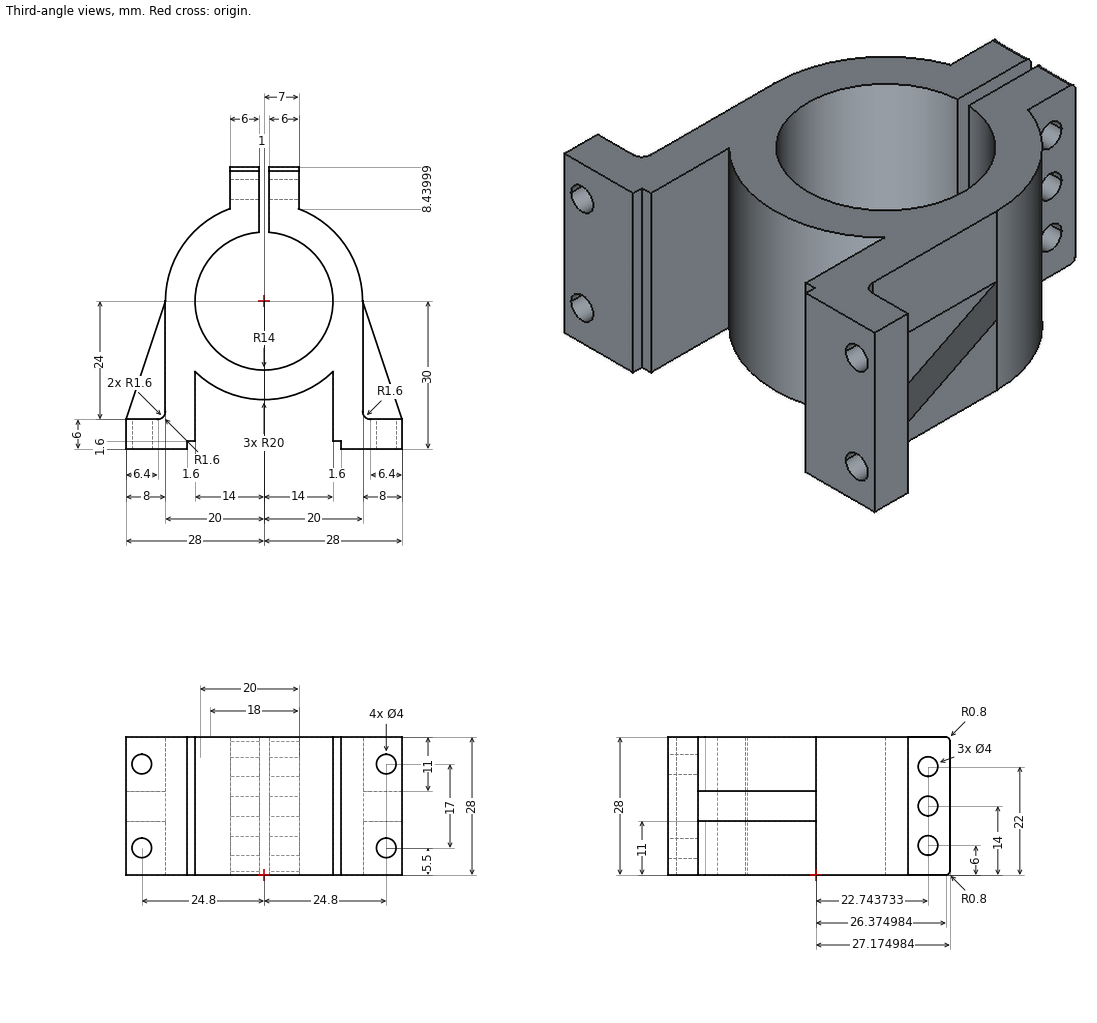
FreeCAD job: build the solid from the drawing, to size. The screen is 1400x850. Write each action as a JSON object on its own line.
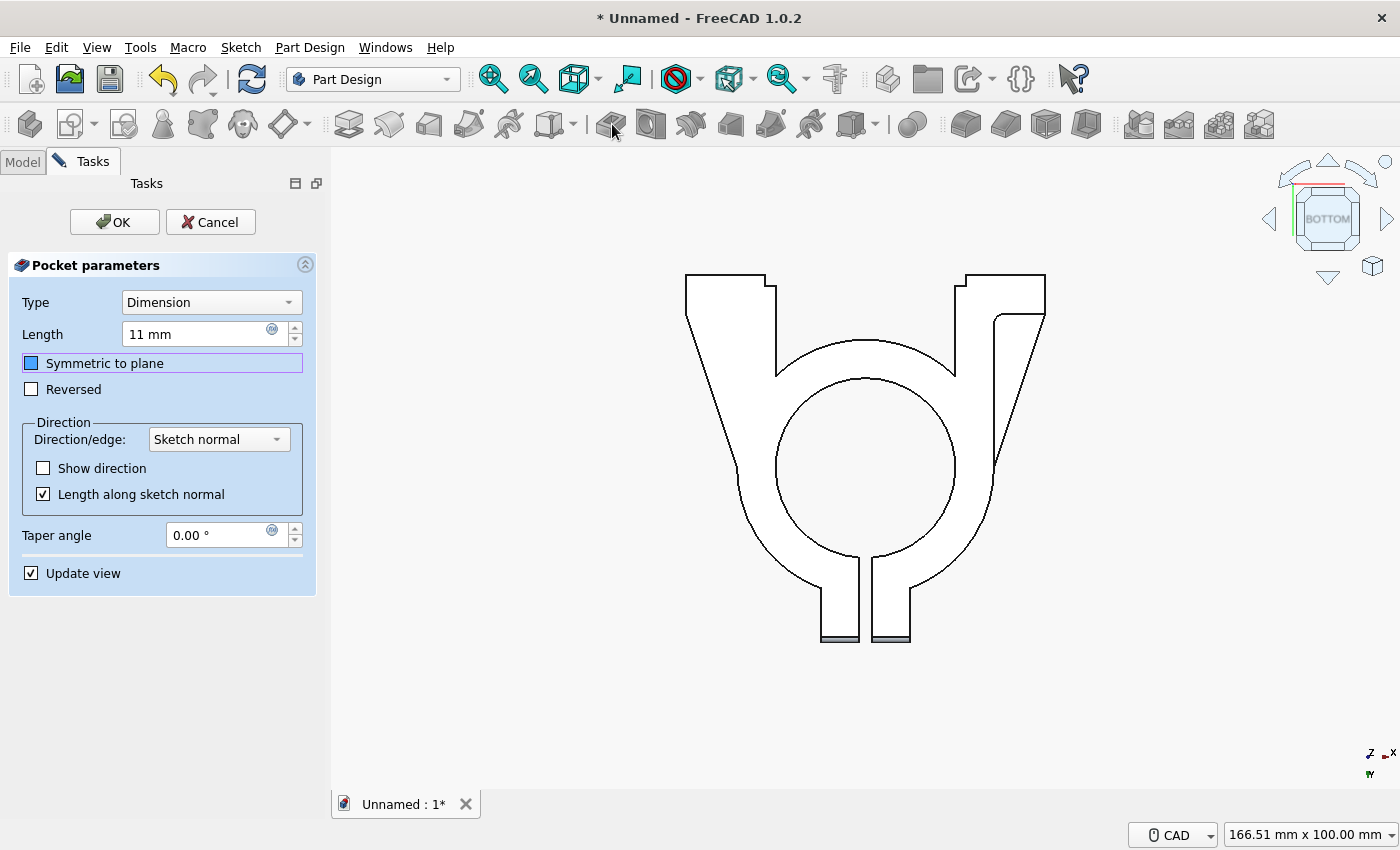
{"action": "left_click", "coordinate": [30, 389]}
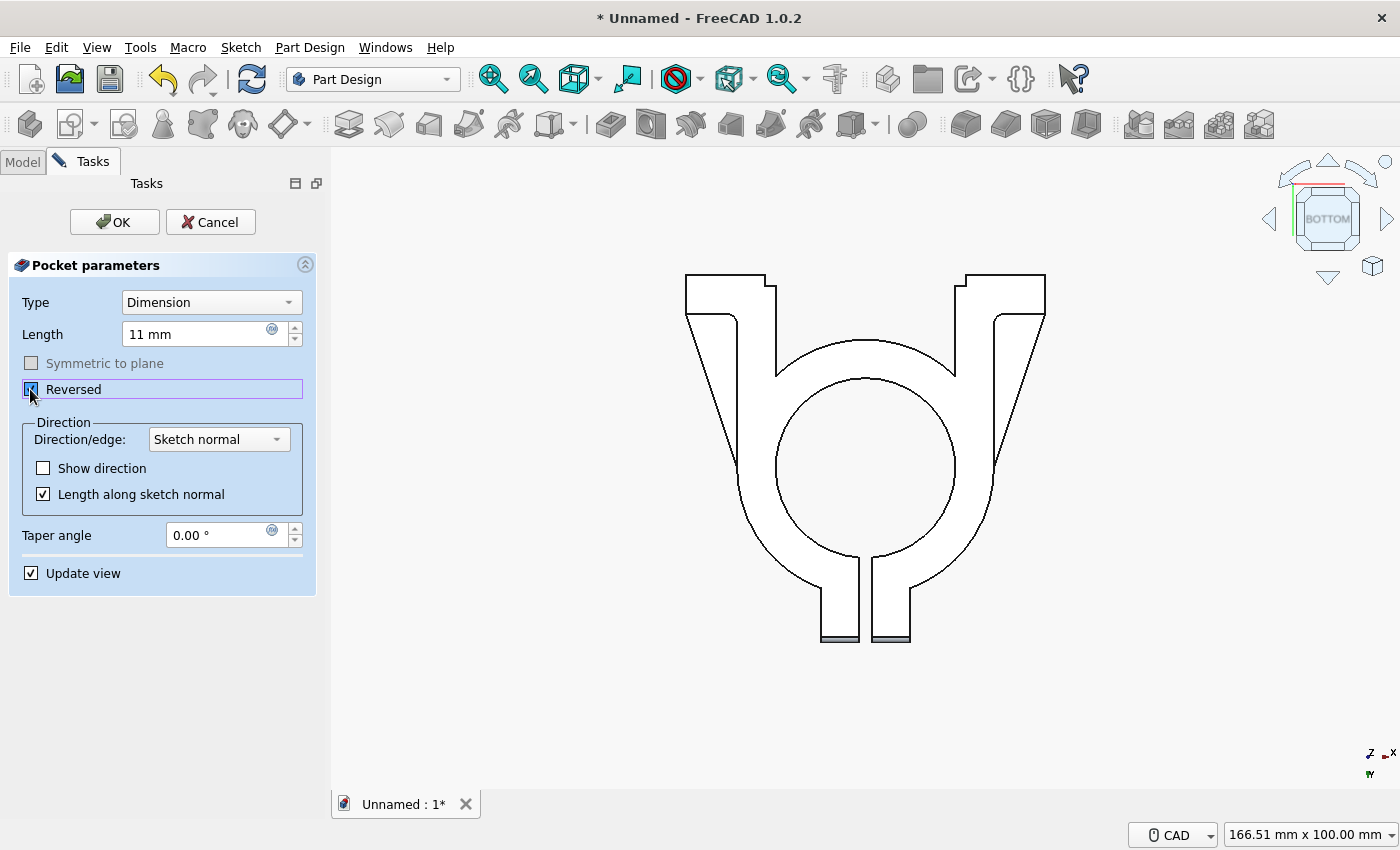
{"action": "left_click", "coordinate": [115, 222]}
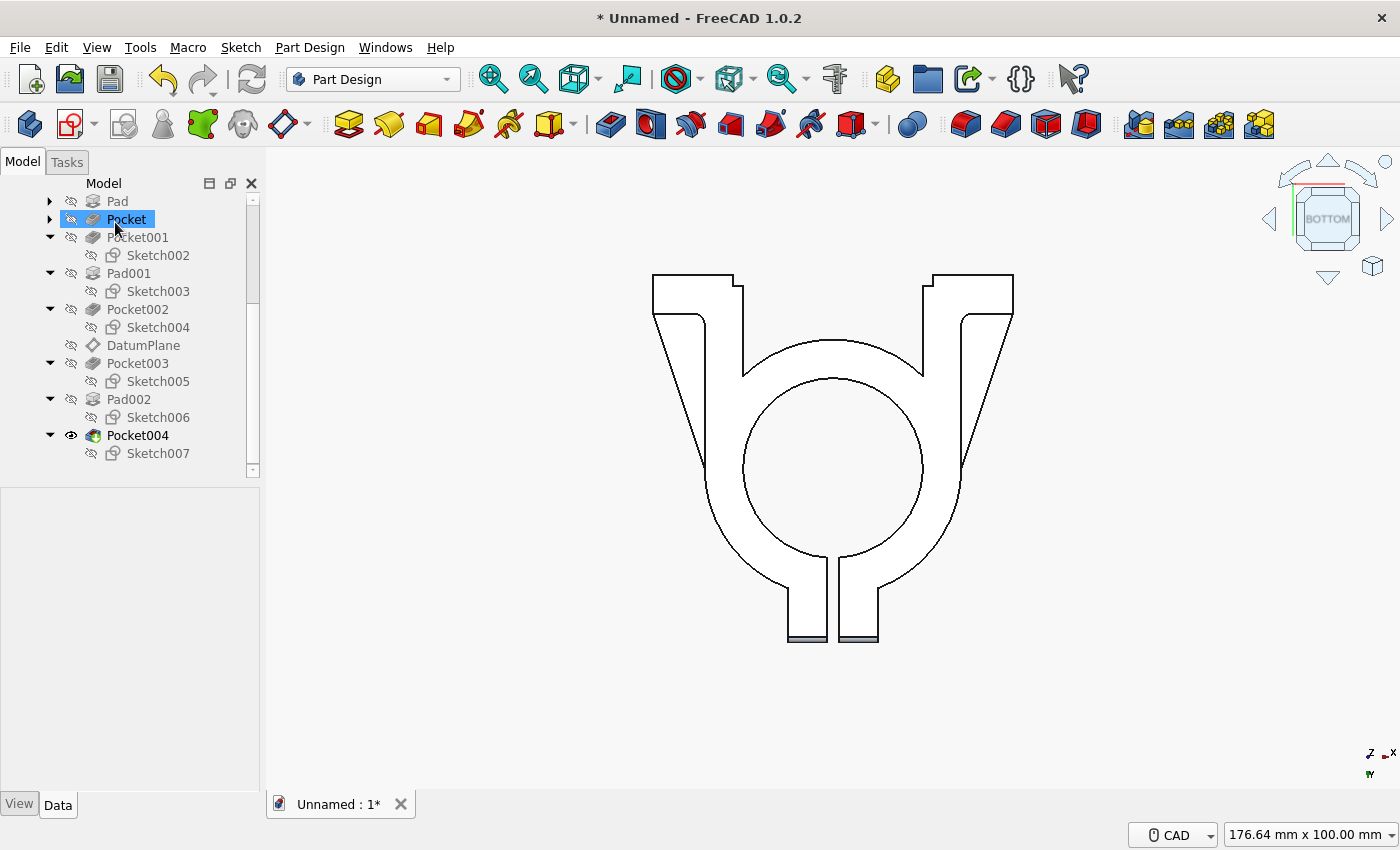
{"action": "key", "text": "0"}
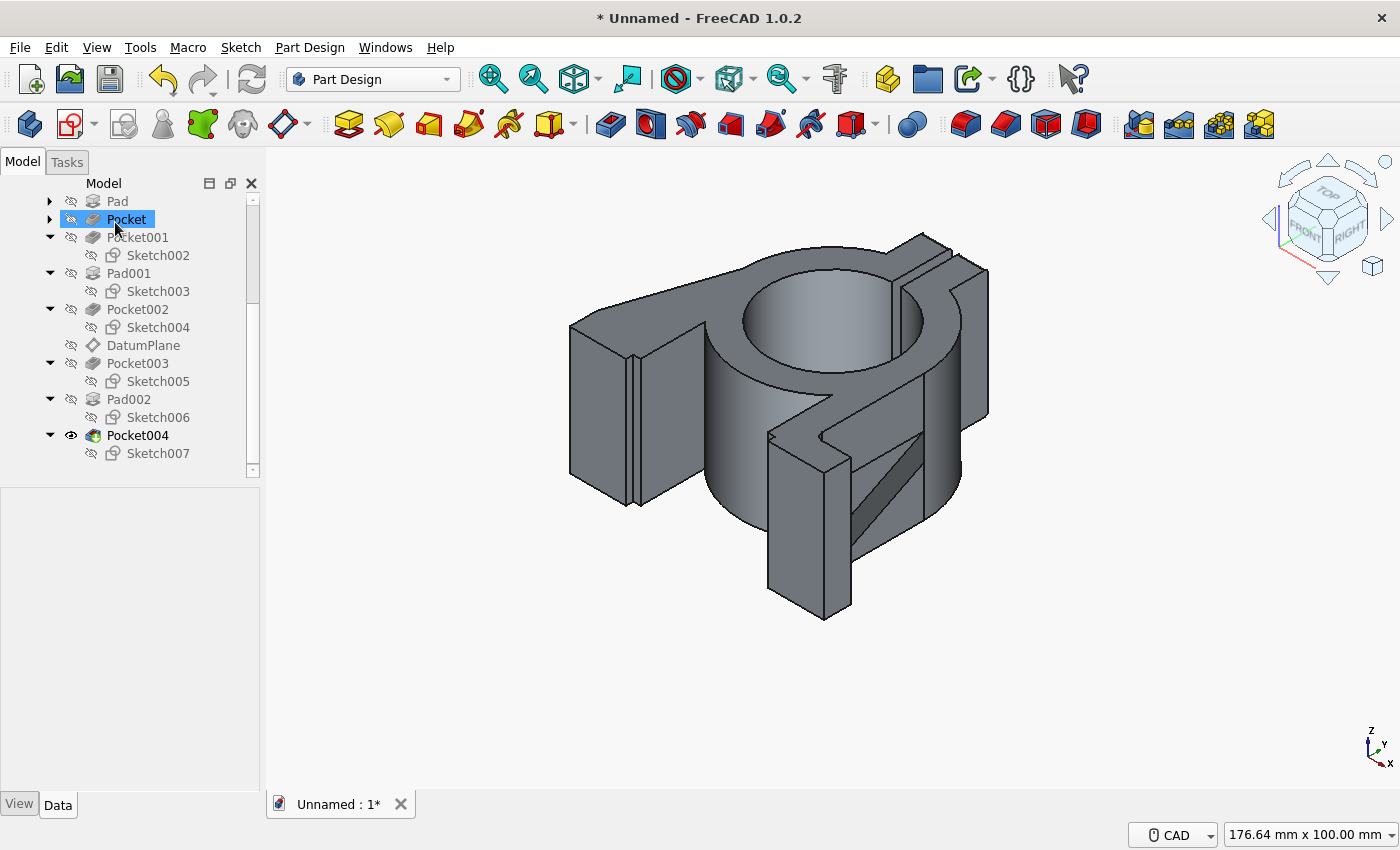
{"action": "left_click", "coordinate": [867, 478]}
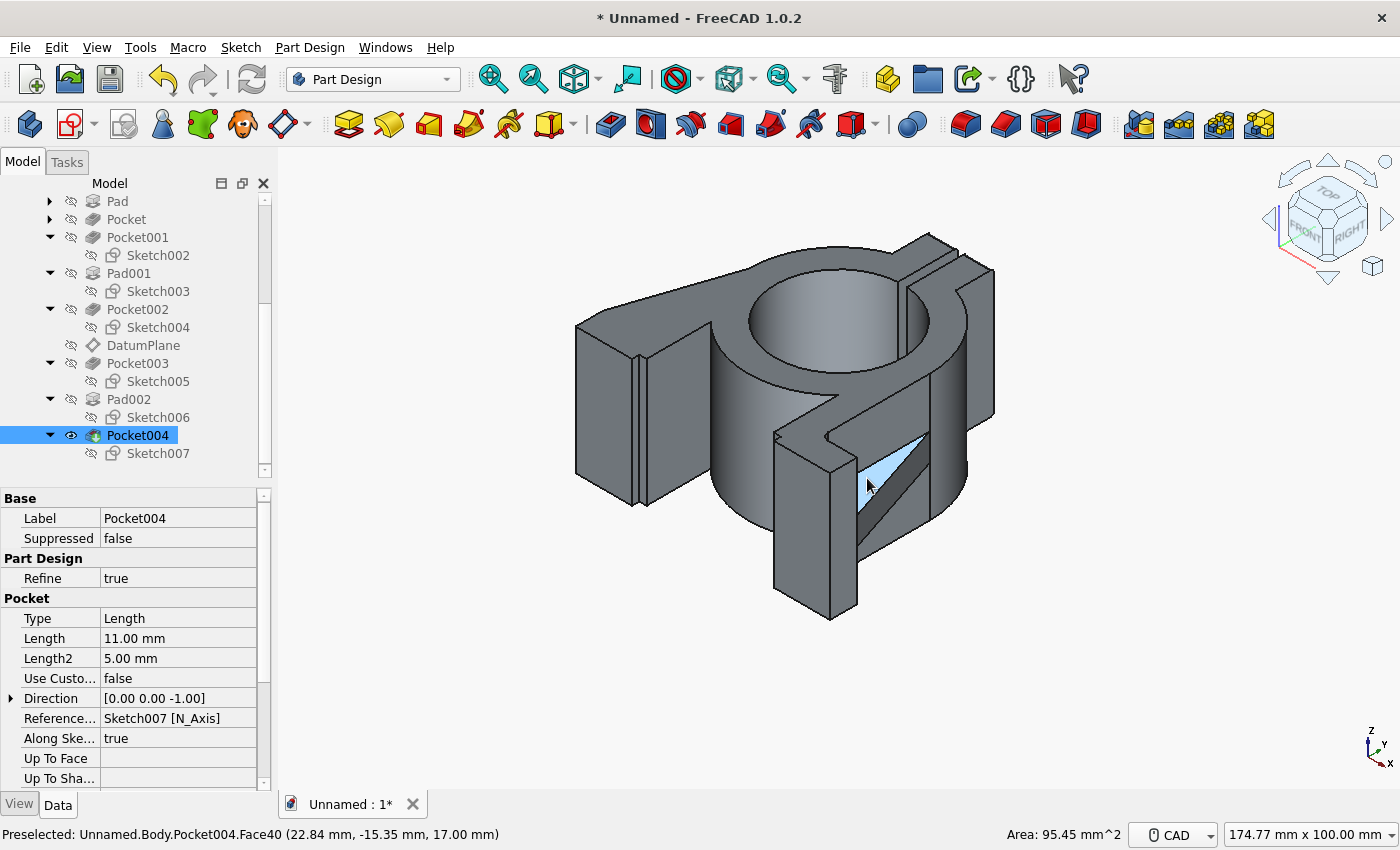
{"action": "left_click", "coordinate": [70, 124]}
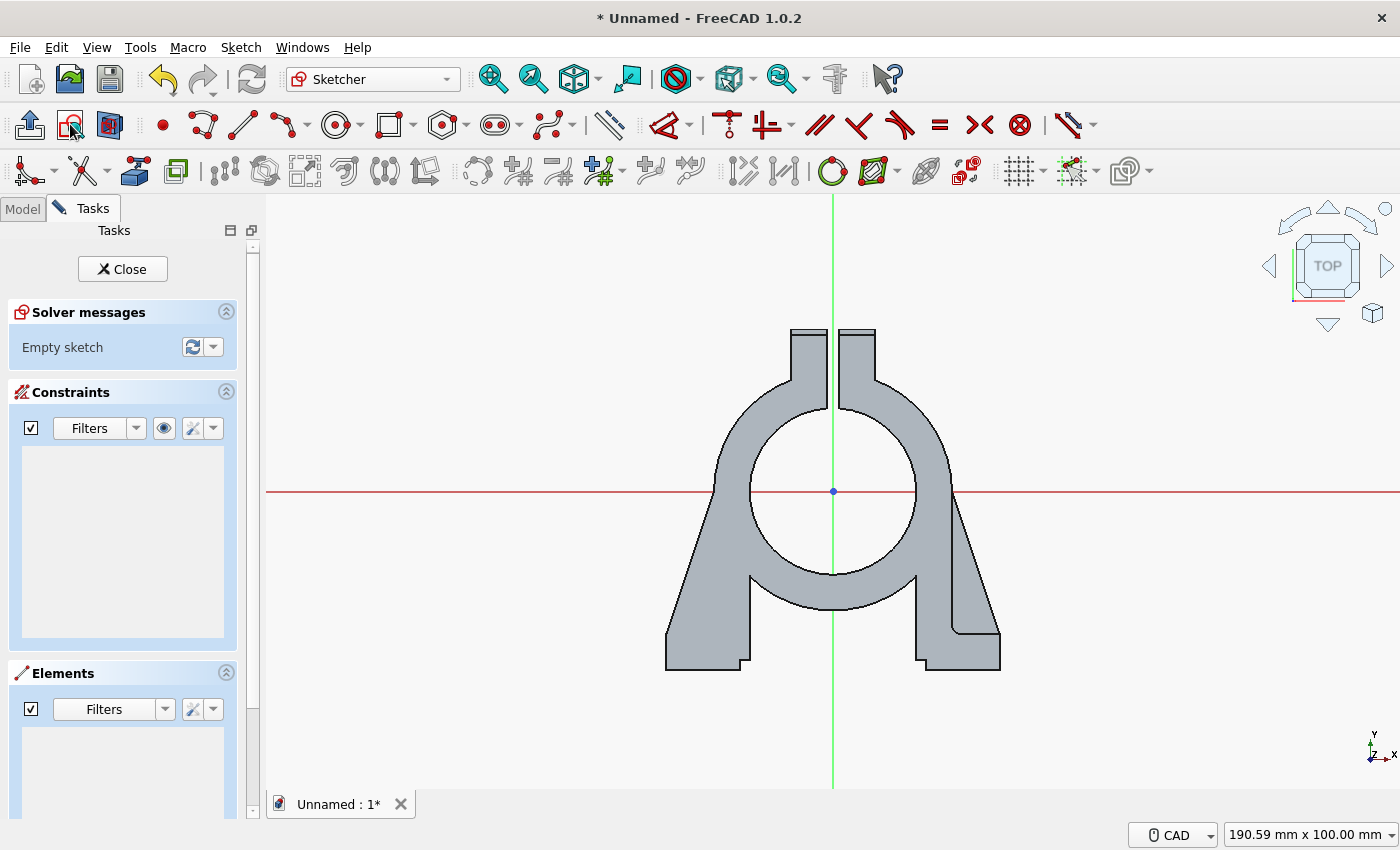
{"action": "scroll", "coordinate": [741, 604], "scroll_direction": "up", "scroll_amount": 5}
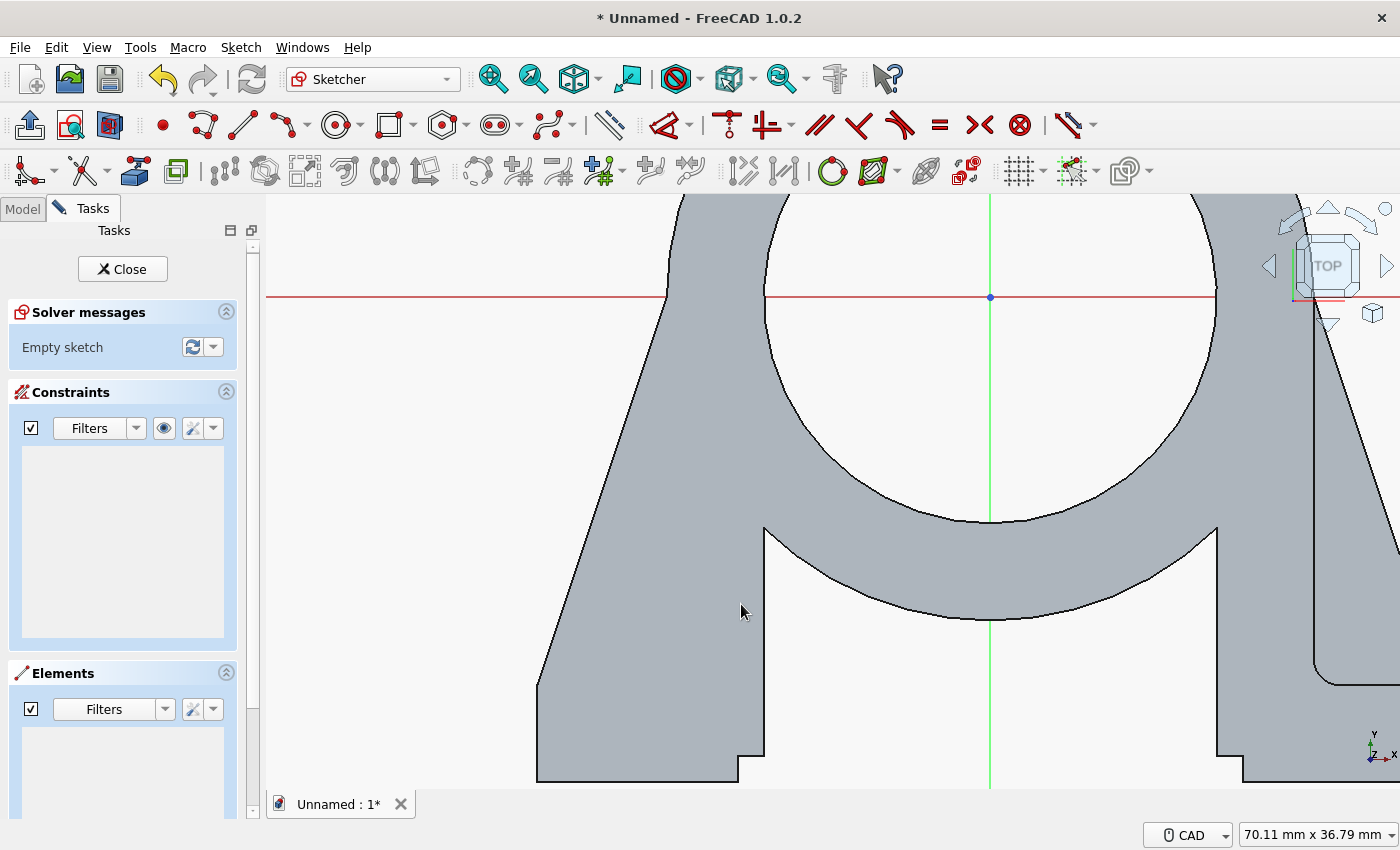
{"action": "left_click", "coordinate": [204, 126]}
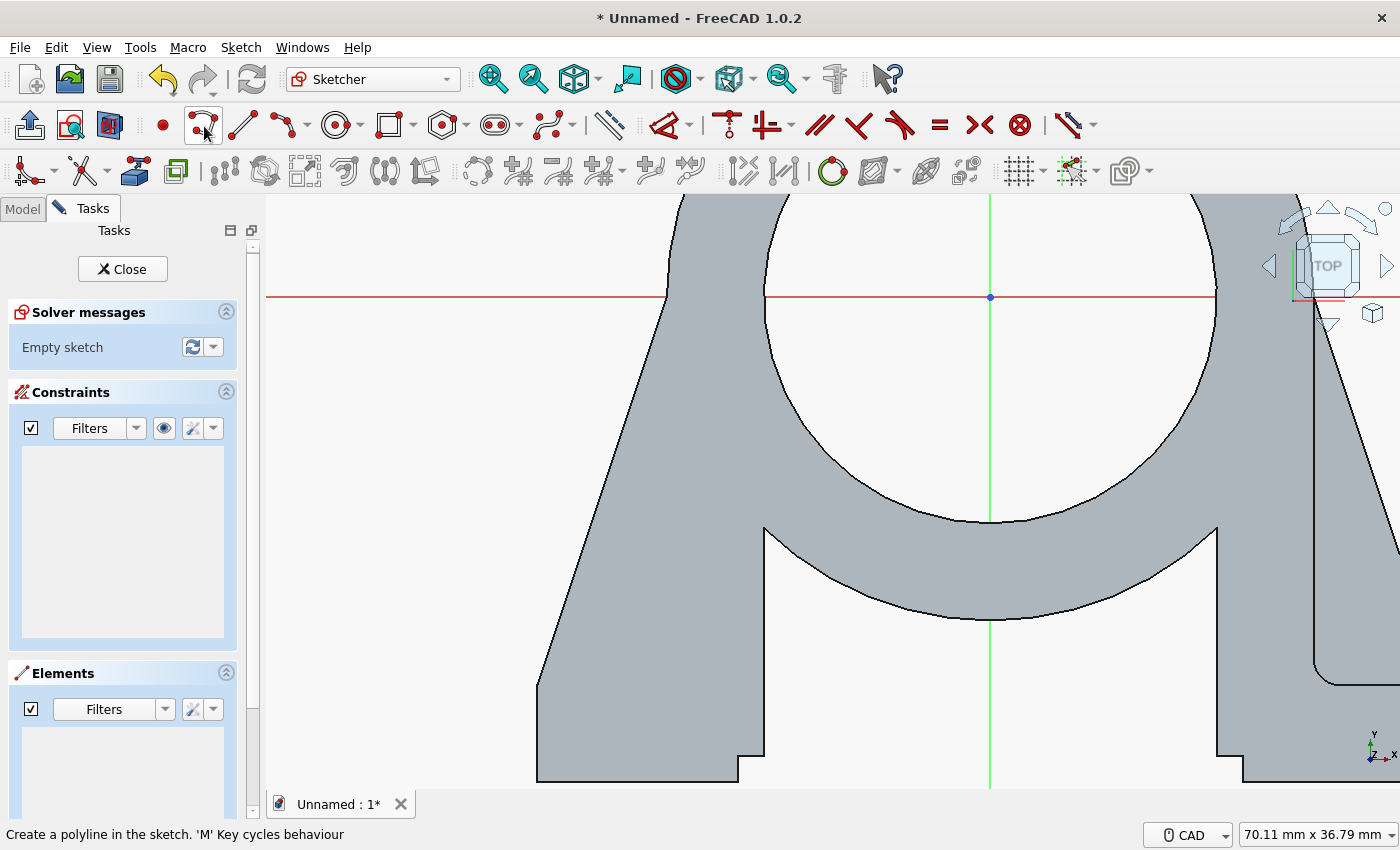
{"action": "left_click", "coordinate": [667, 659]}
{"action": "left_click", "coordinate": [667, 297]}
{"action": "left_click", "coordinate": [537, 685]}
{"action": "left_click", "coordinate": [641, 685]}
{"action": "right_click", "coordinate": [641, 685]}